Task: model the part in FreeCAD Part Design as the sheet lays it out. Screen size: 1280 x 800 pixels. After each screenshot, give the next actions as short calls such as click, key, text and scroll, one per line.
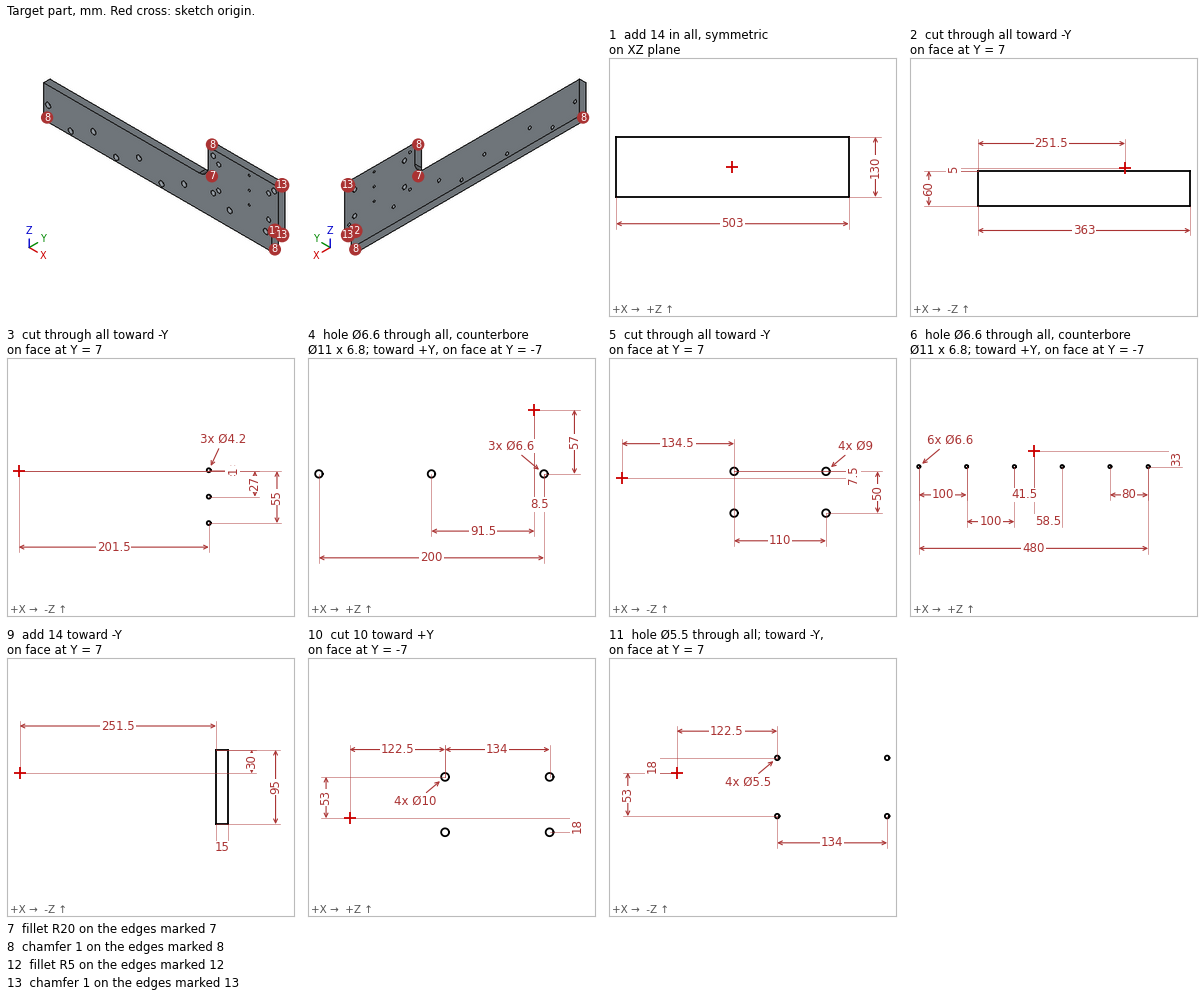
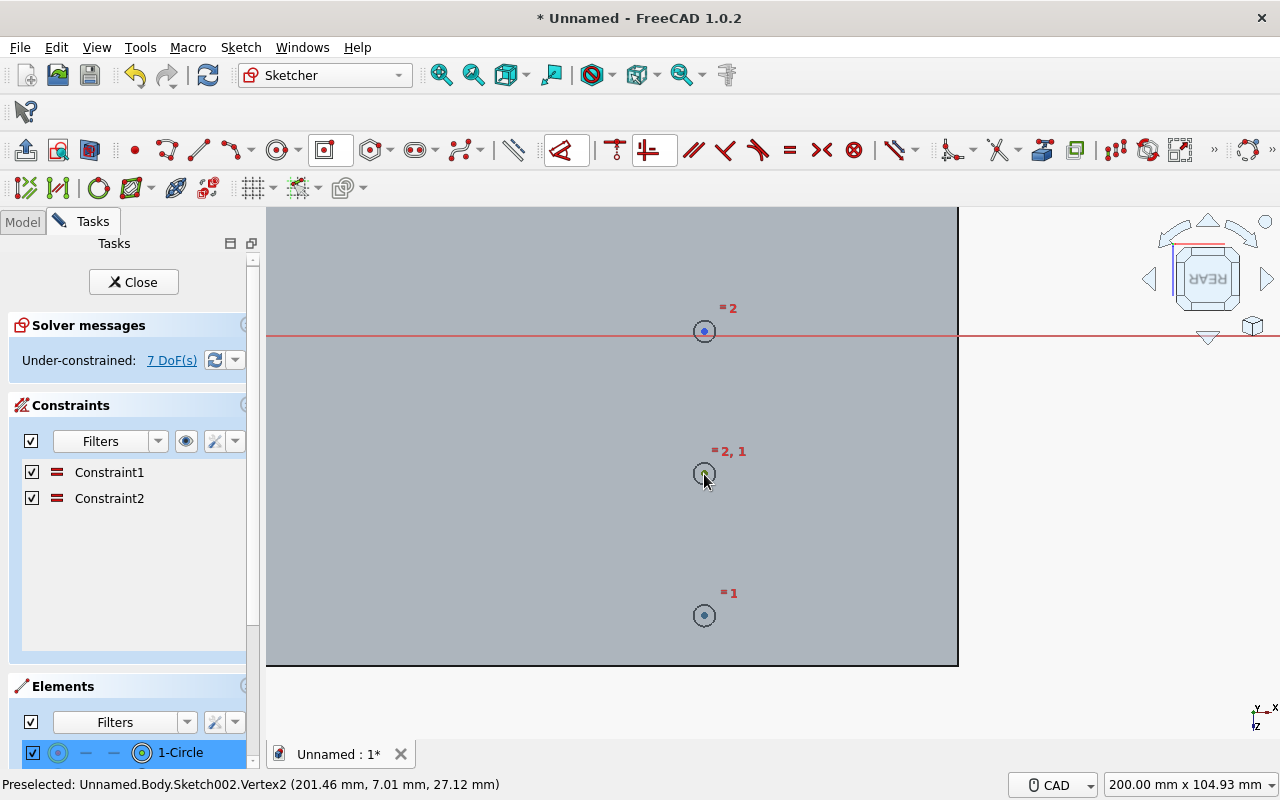
key(v)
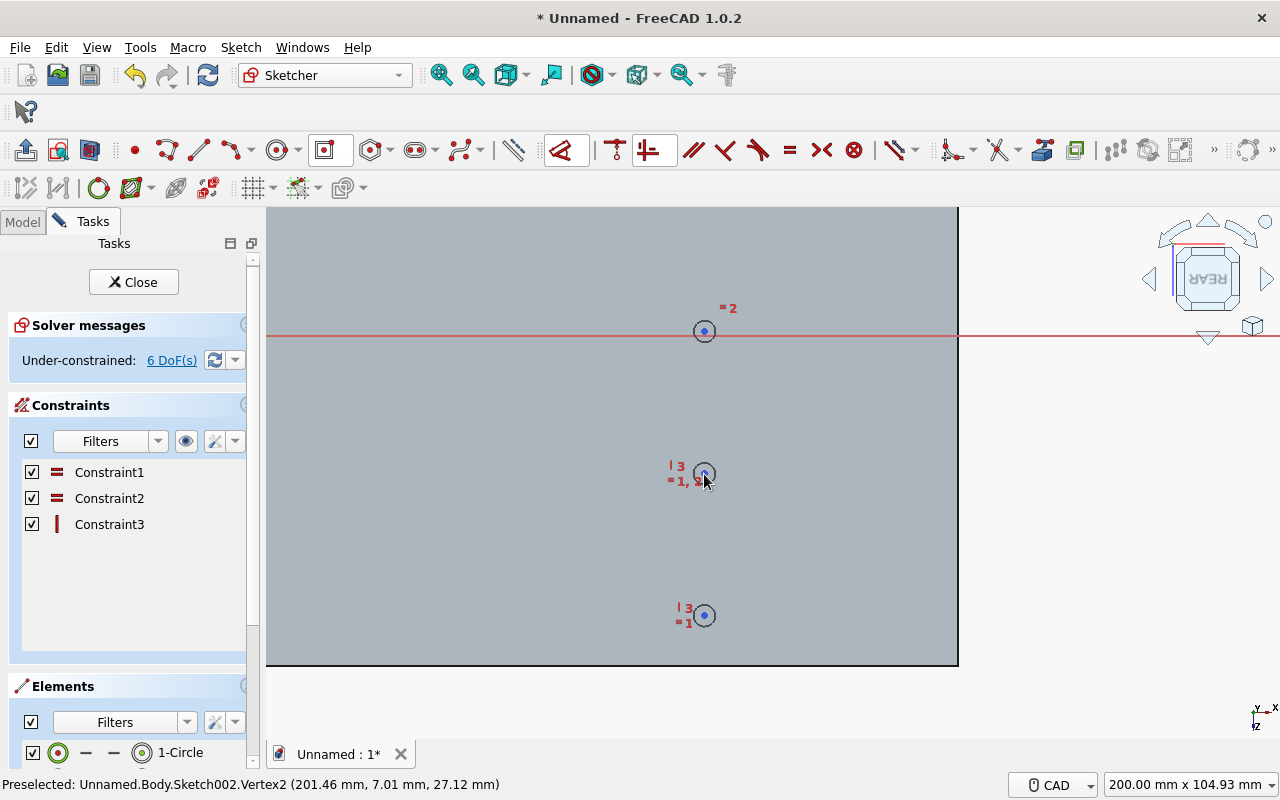
click(704, 474)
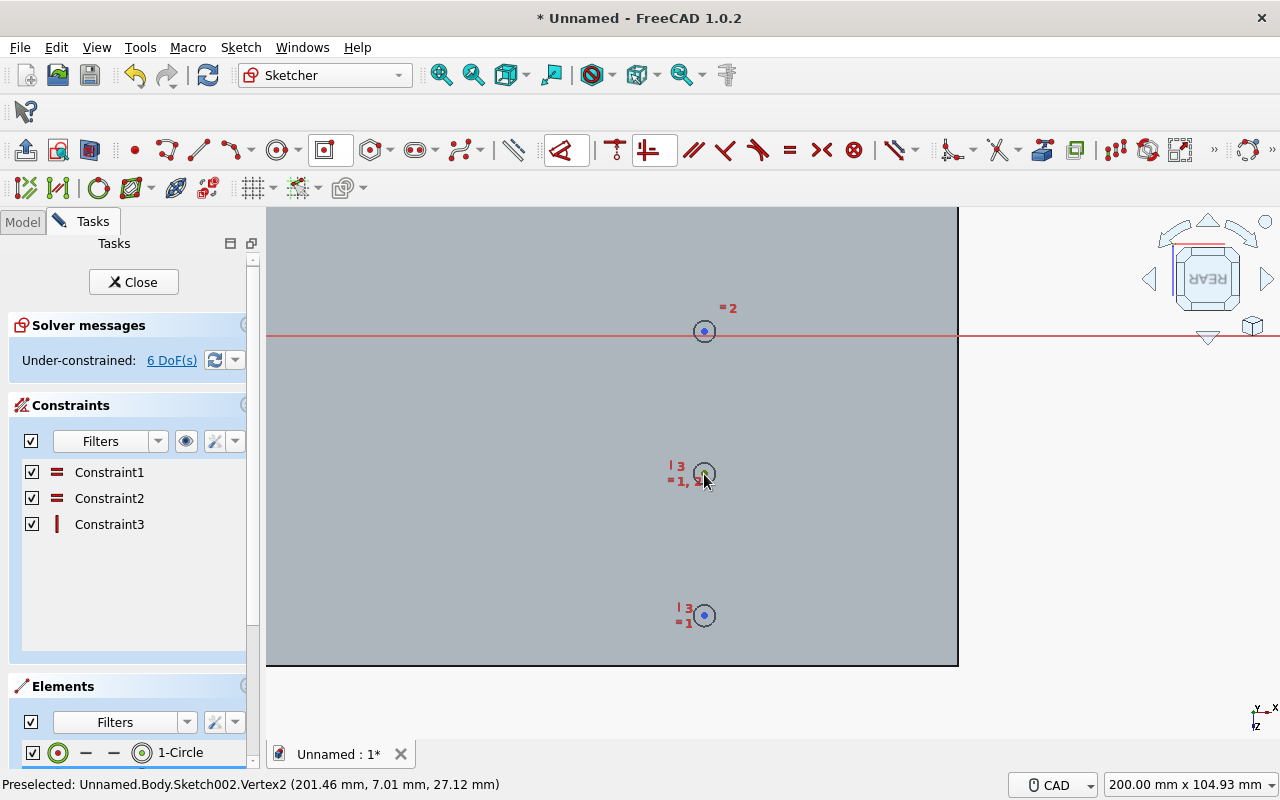
click(705, 331)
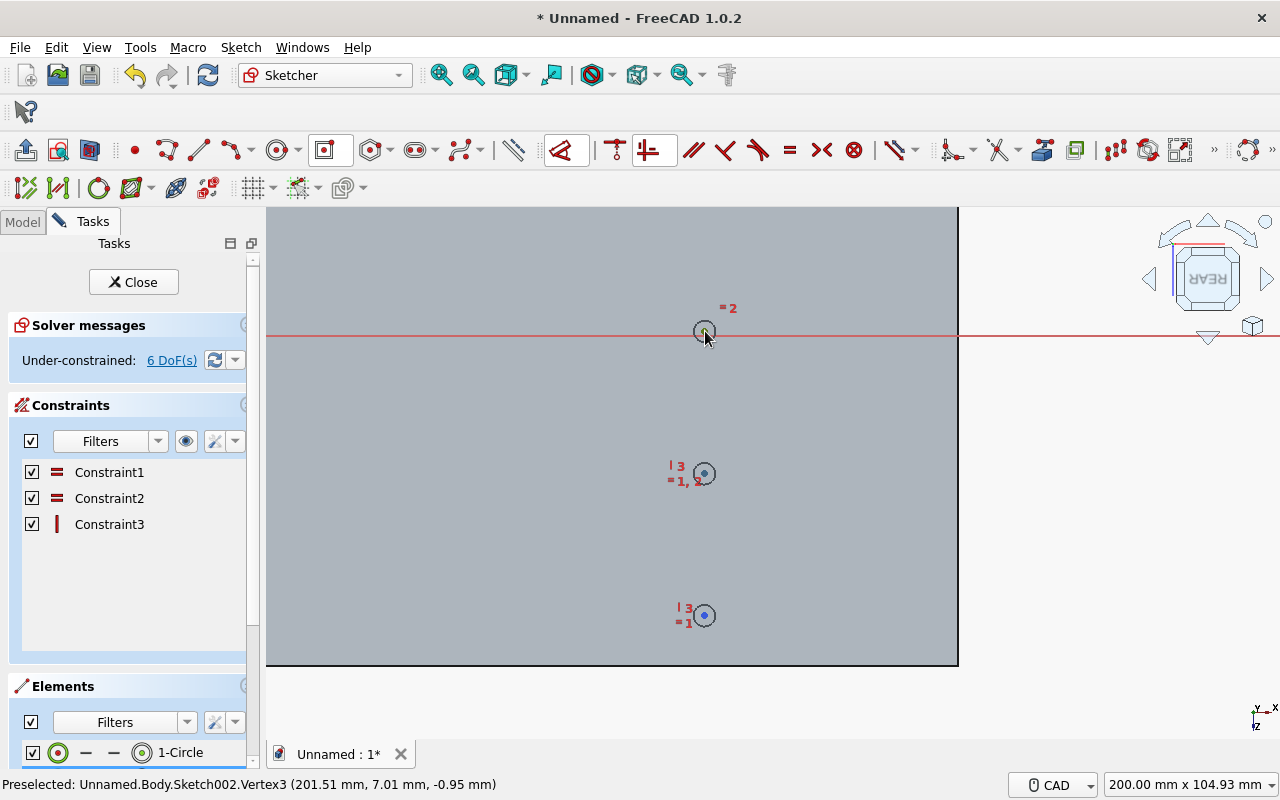
key(v)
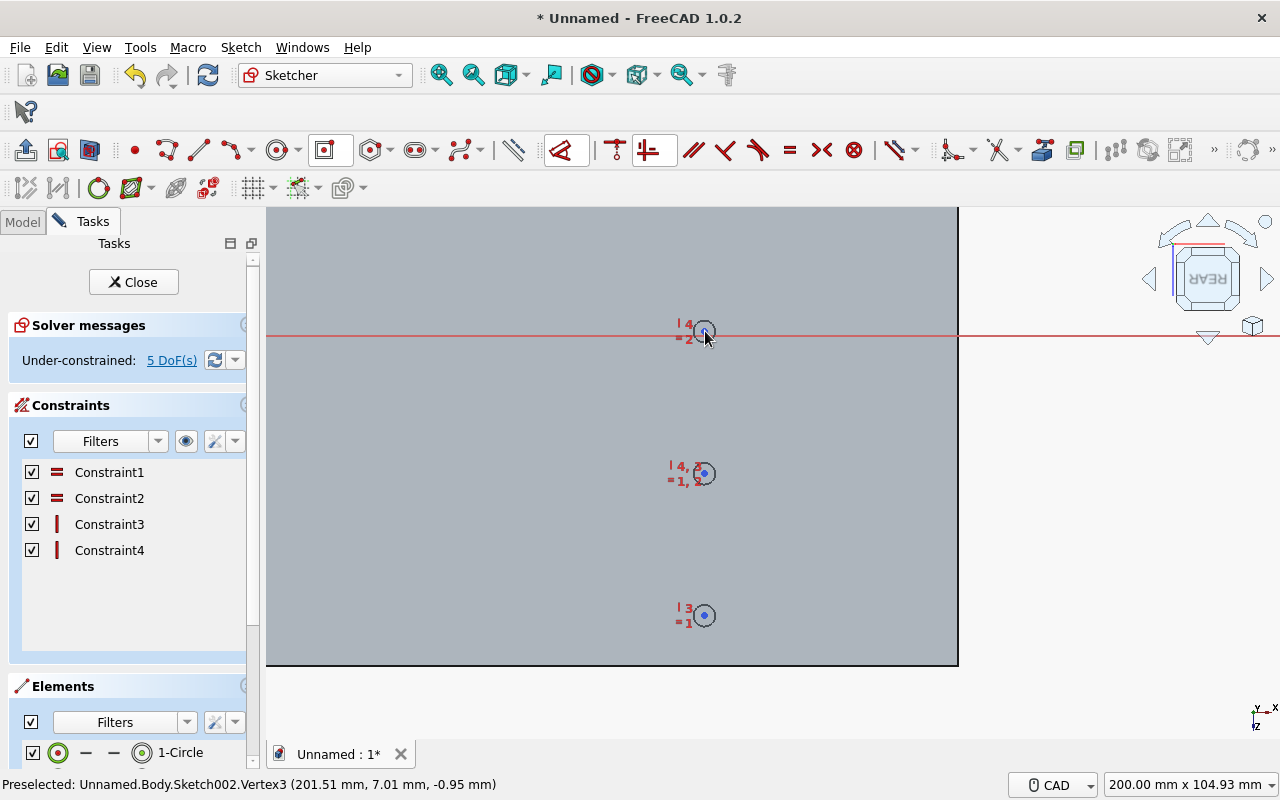
scroll(712, 608, up, 4)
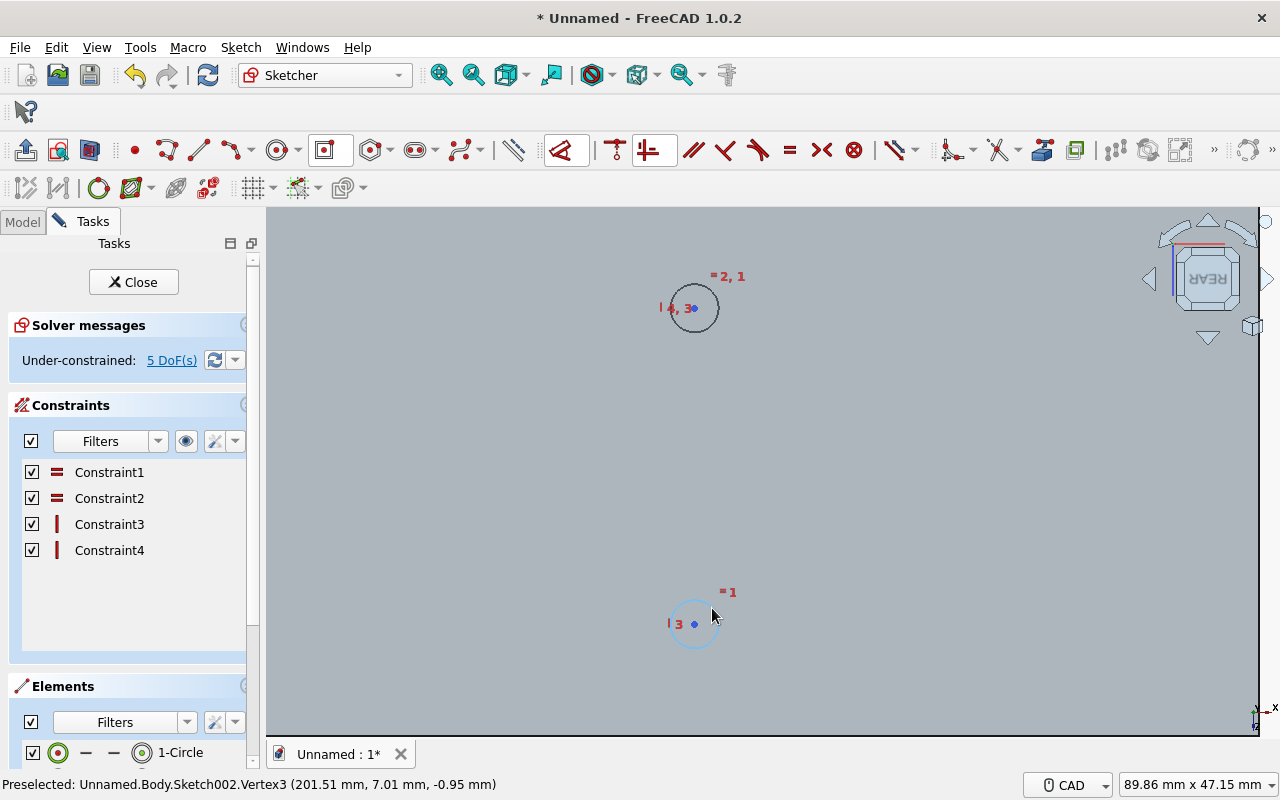
click(712, 607)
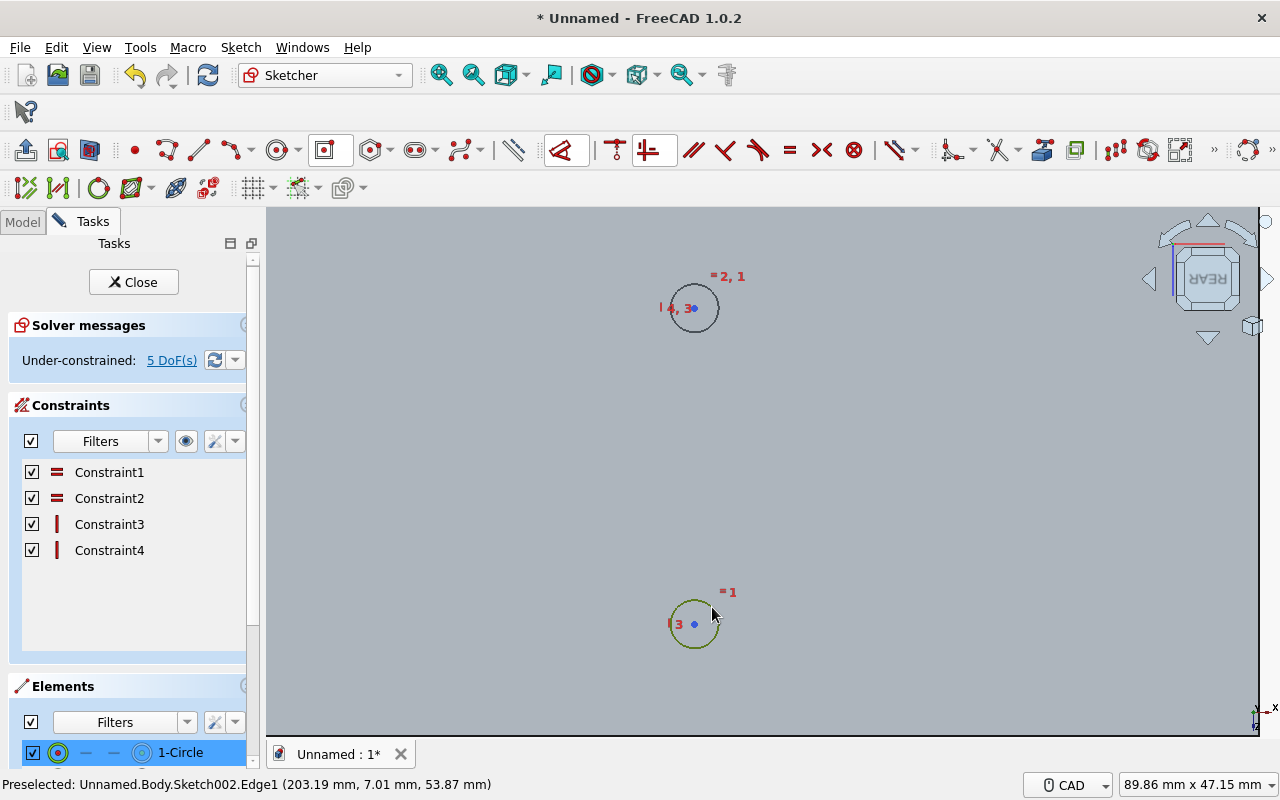
key(k)
key(o)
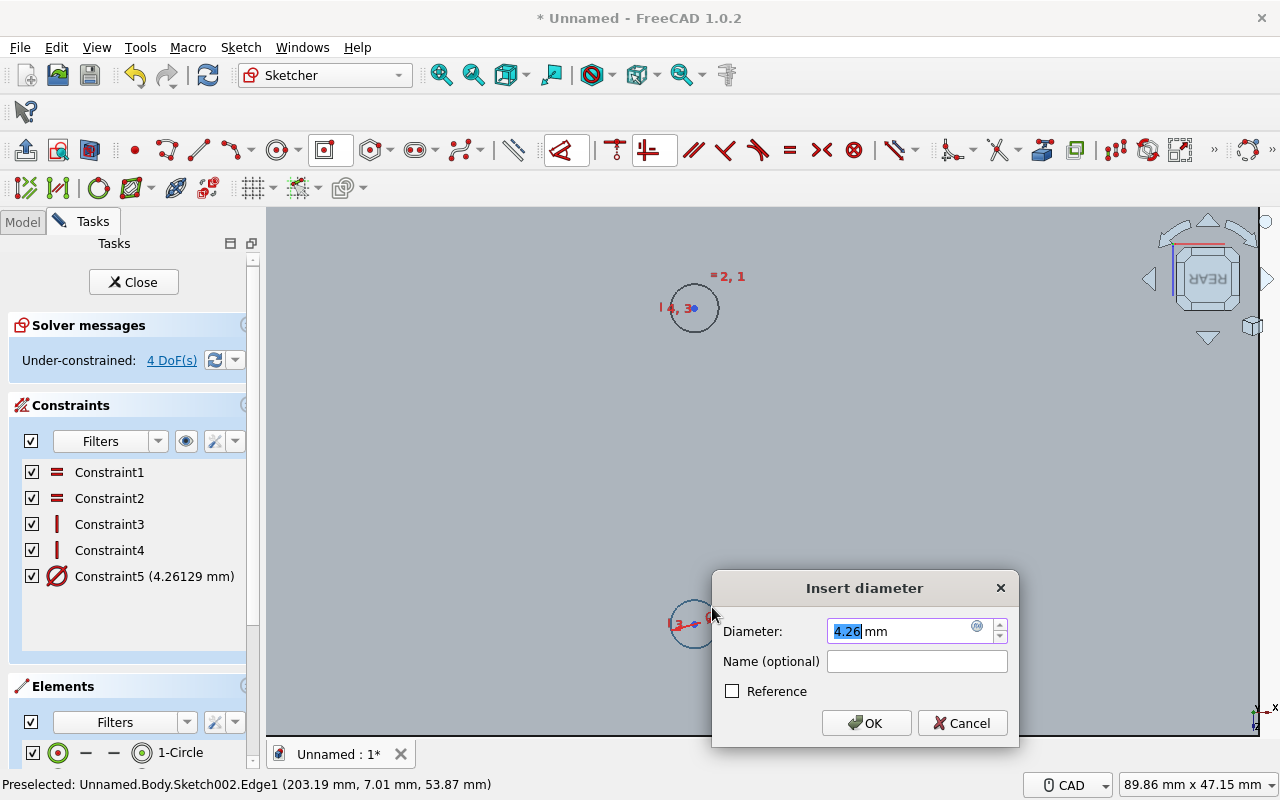
text(4.2)
key(Return)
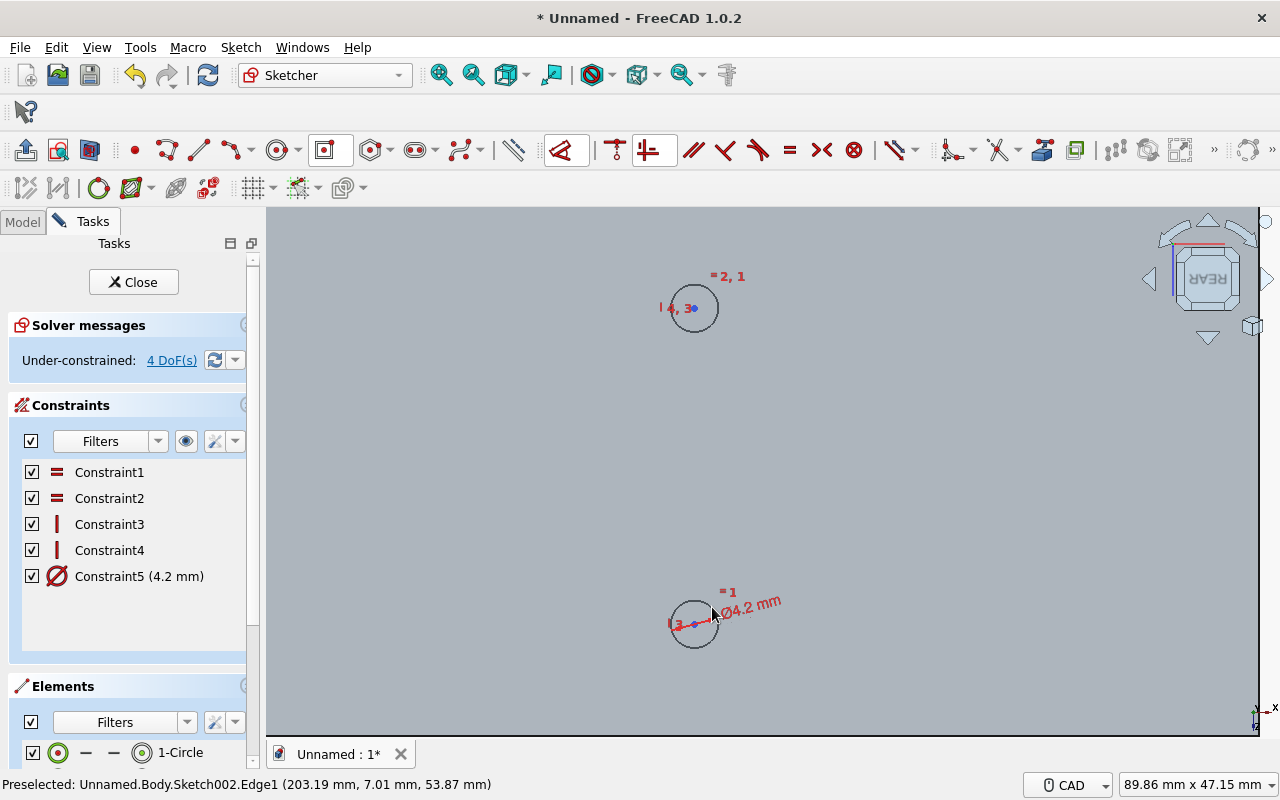
scroll(712, 608, down, 4)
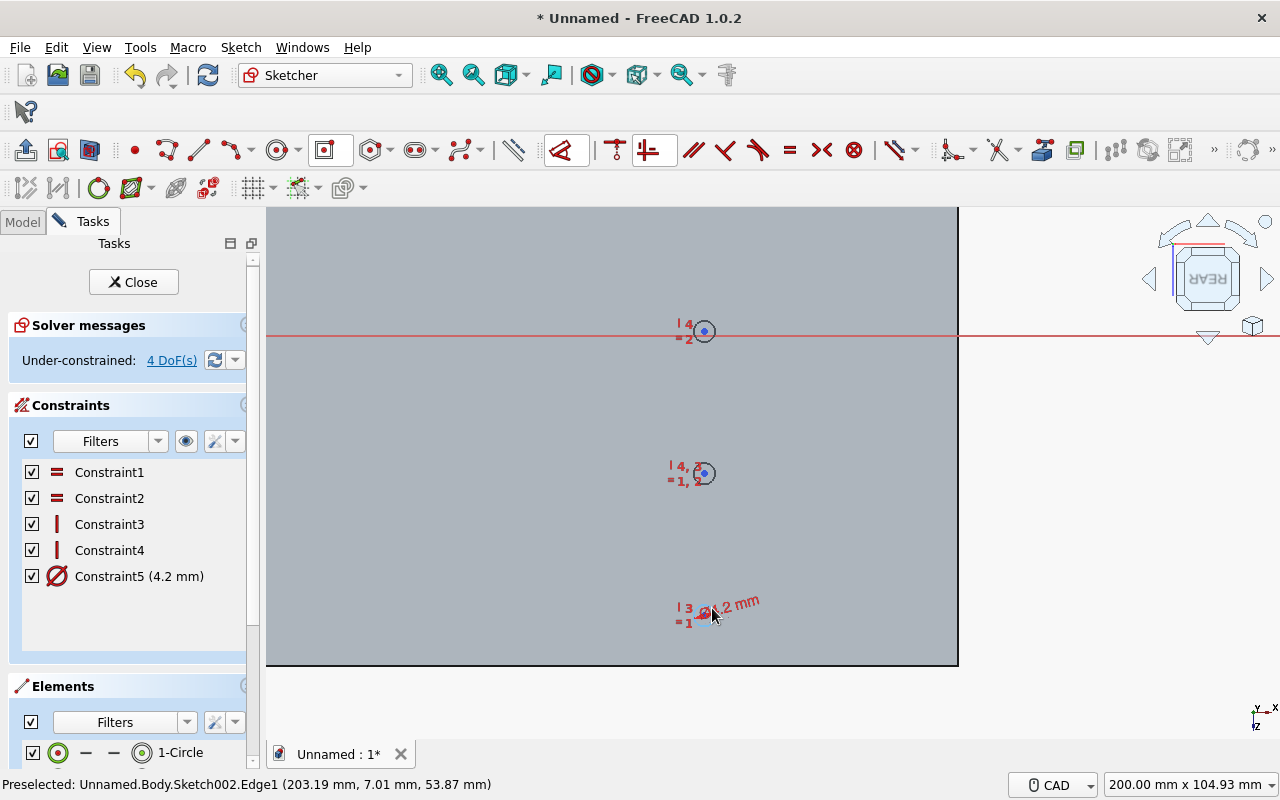
scroll(704, 331, up, 11)